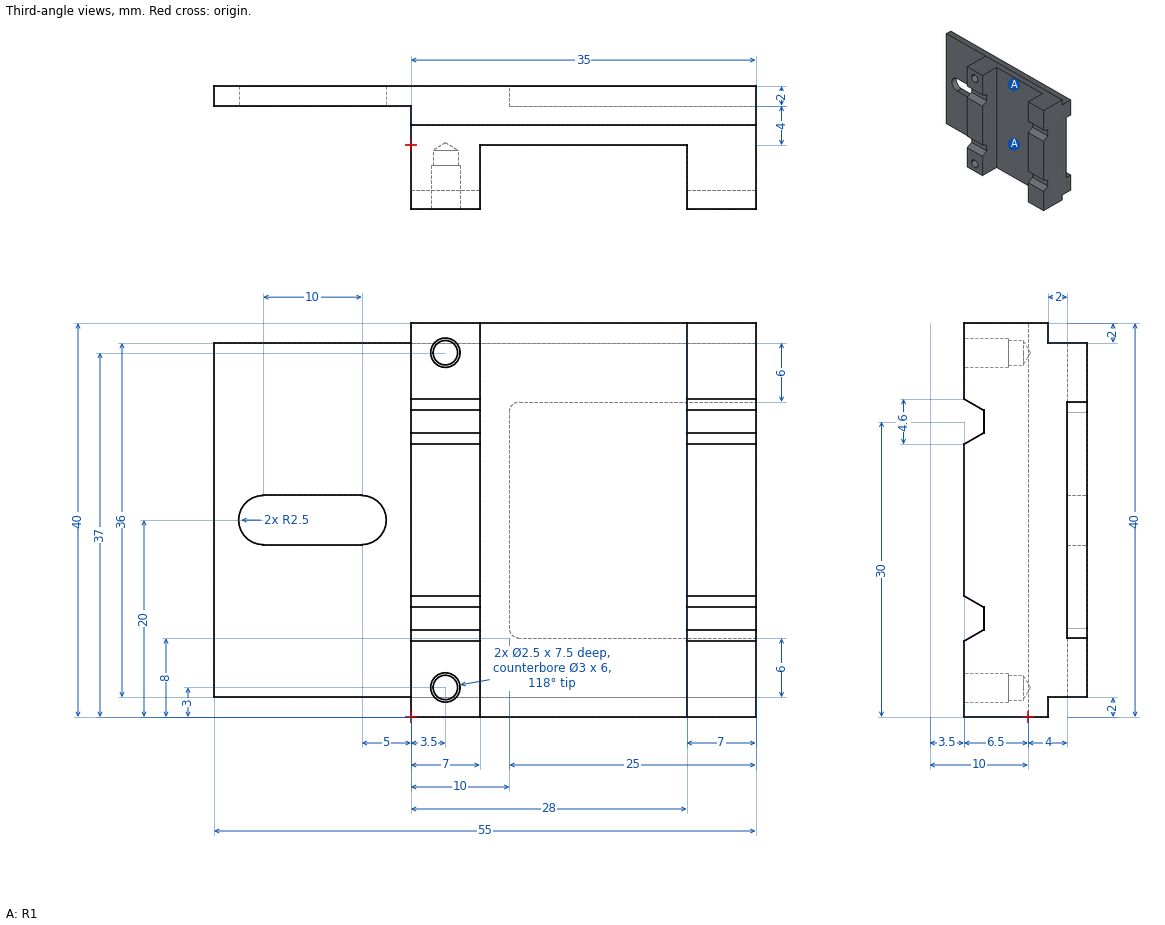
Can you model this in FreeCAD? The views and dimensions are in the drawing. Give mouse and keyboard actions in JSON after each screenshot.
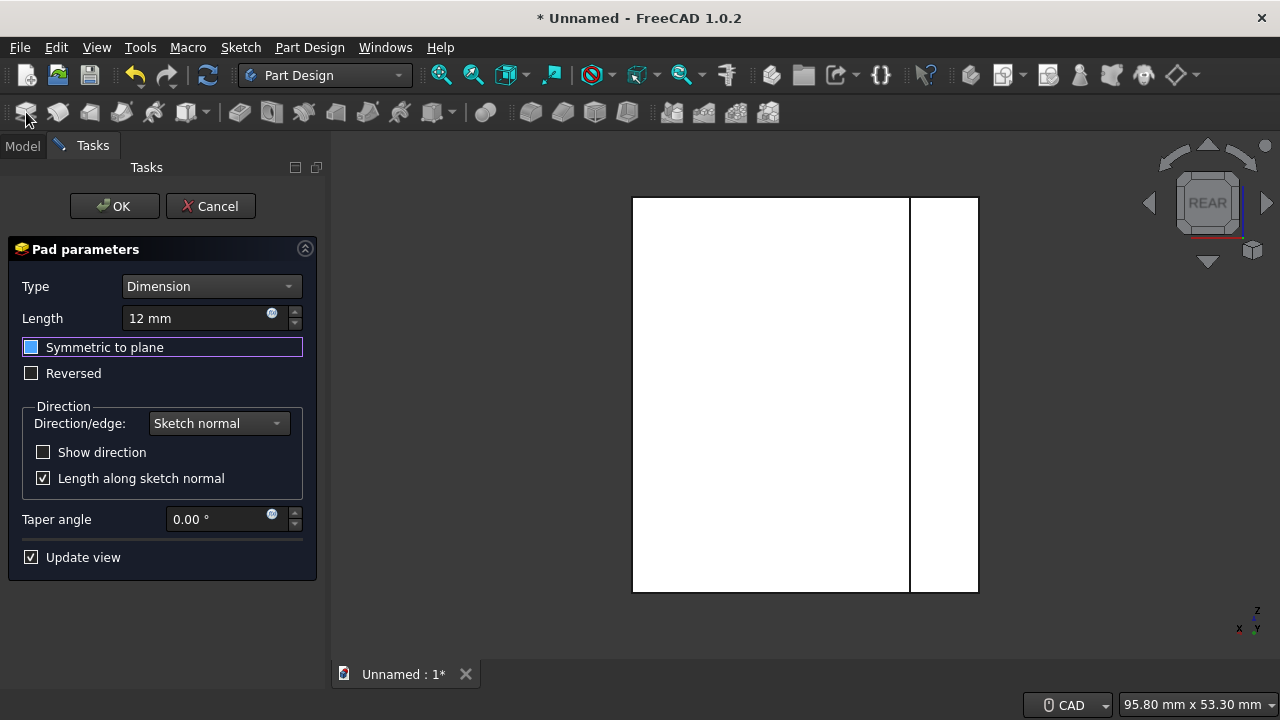
{"action": "left_click", "coordinate": [30, 373]}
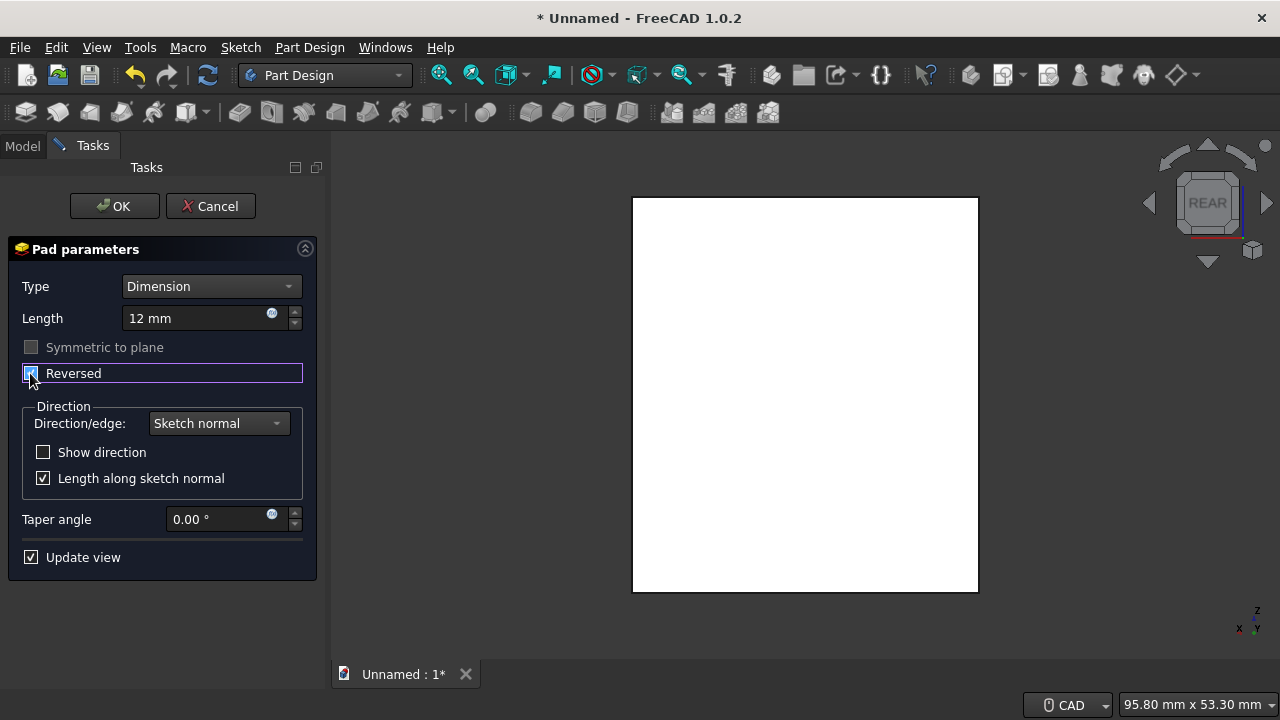
{"action": "left_click", "coordinate": [115, 206]}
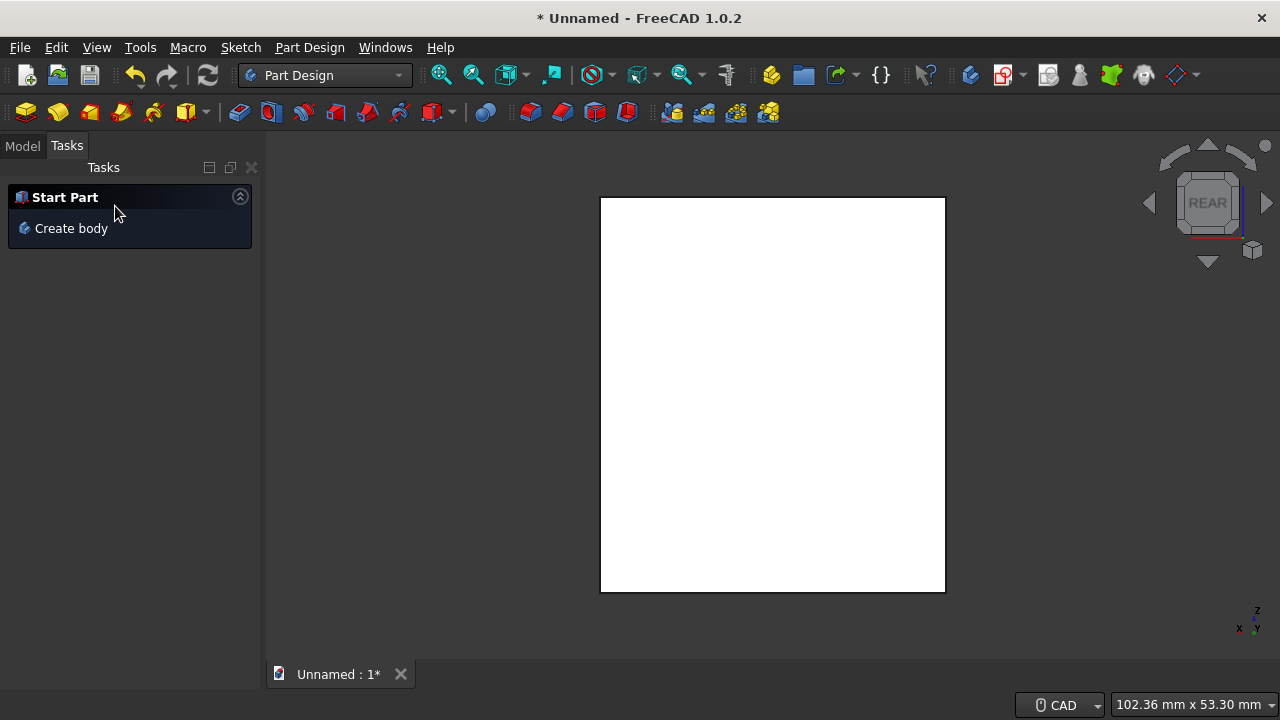
{"action": "key", "text": "0"}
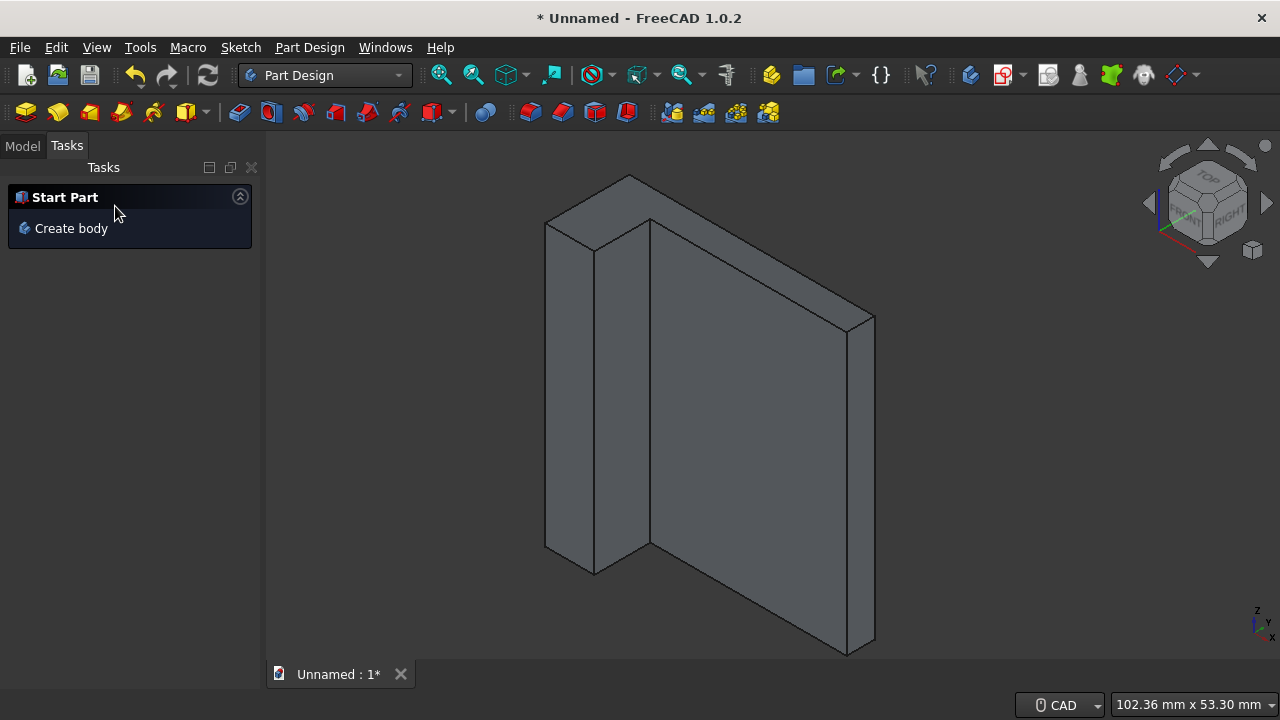
{"action": "left_click", "coordinate": [442, 76]}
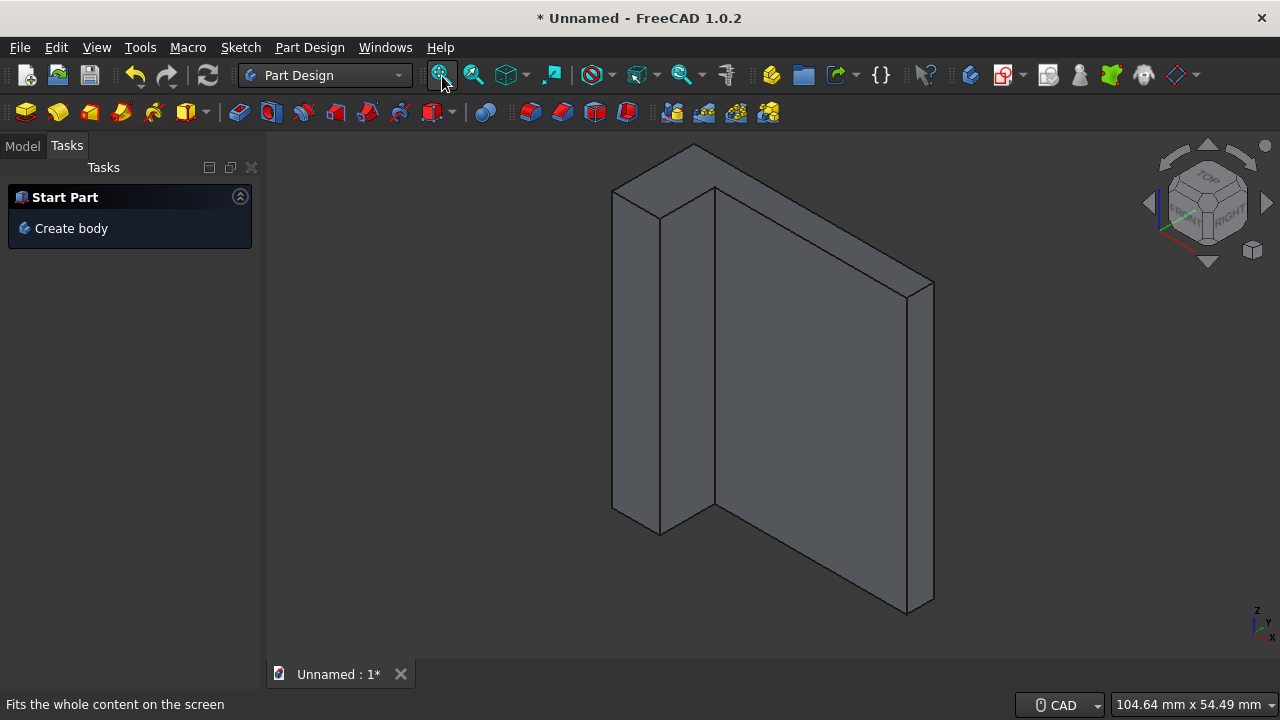
{"action": "left_click", "coordinate": [636, 272]}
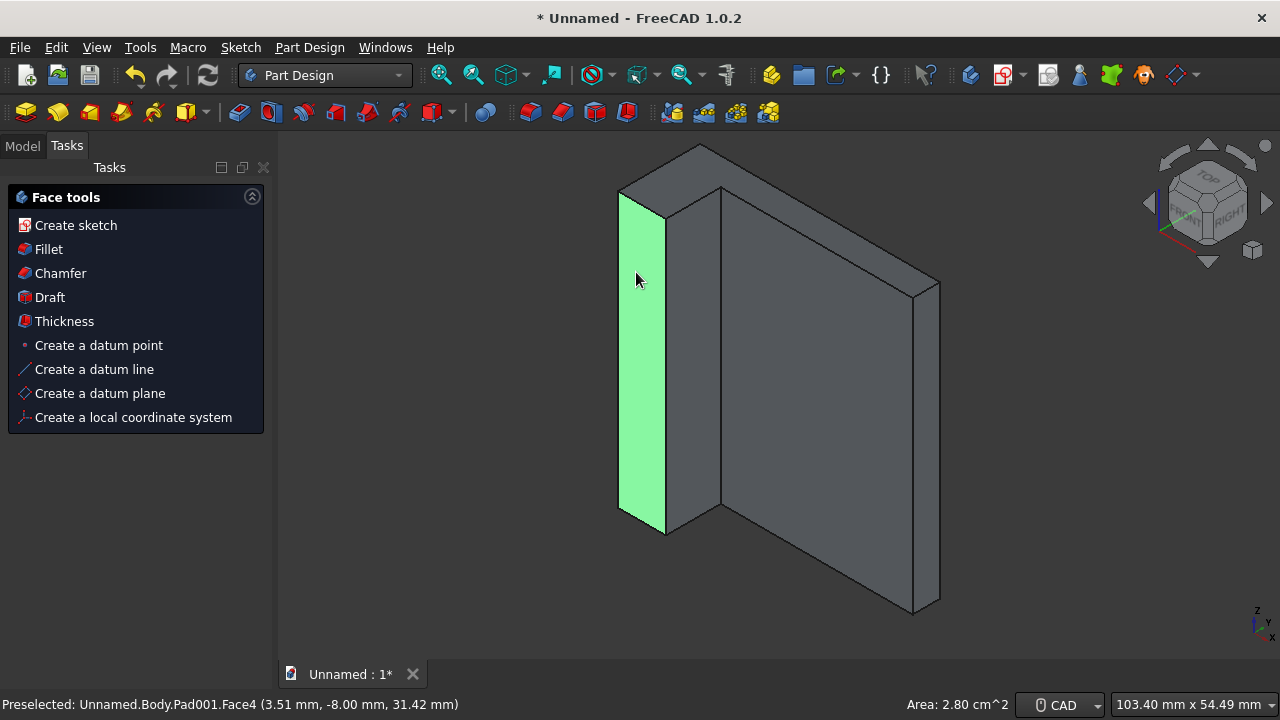
{"action": "left_click", "coordinate": [1004, 76]}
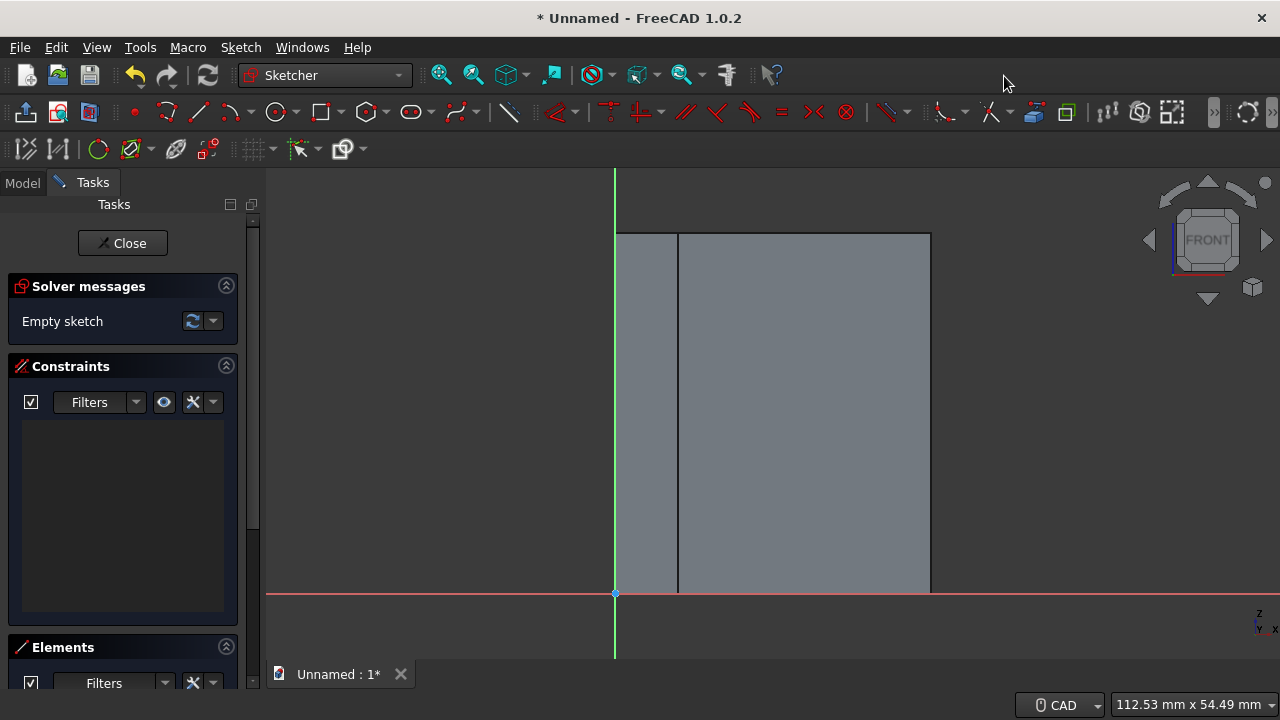
{"action": "left_click", "coordinate": [276, 112]}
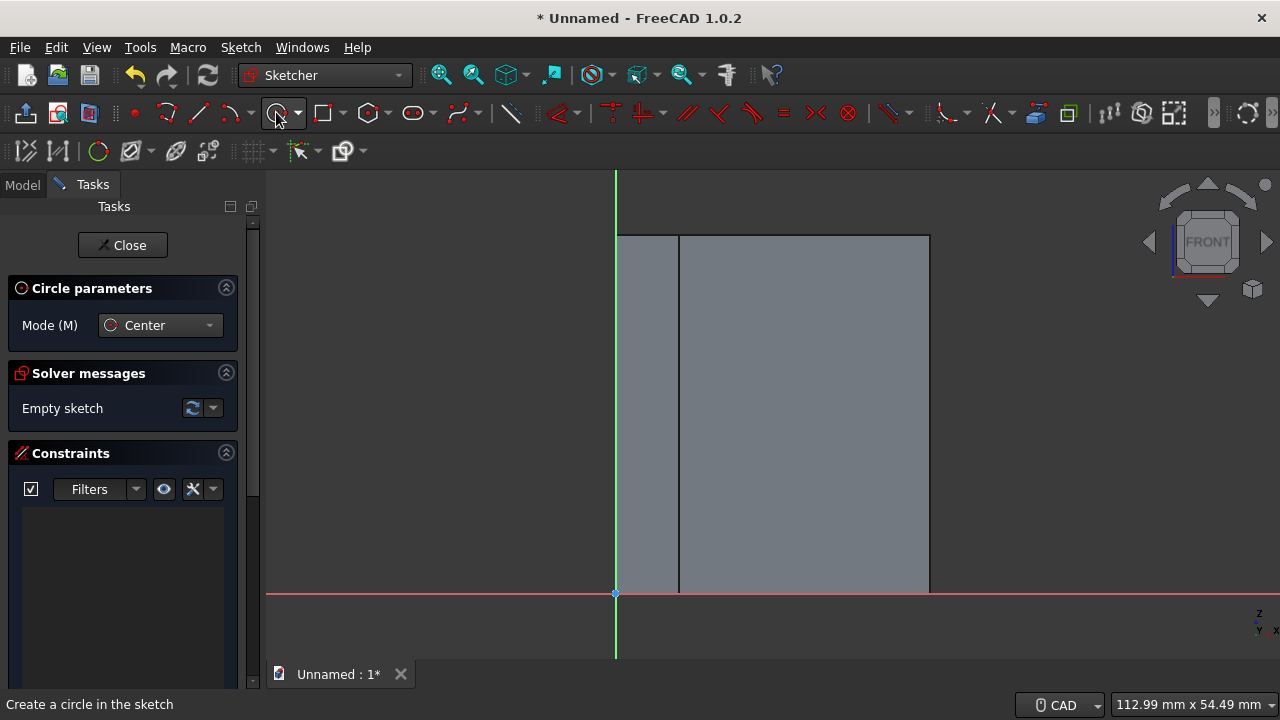
{"action": "scroll", "coordinate": [647, 567], "scroll_direction": "up", "scroll_amount": 4}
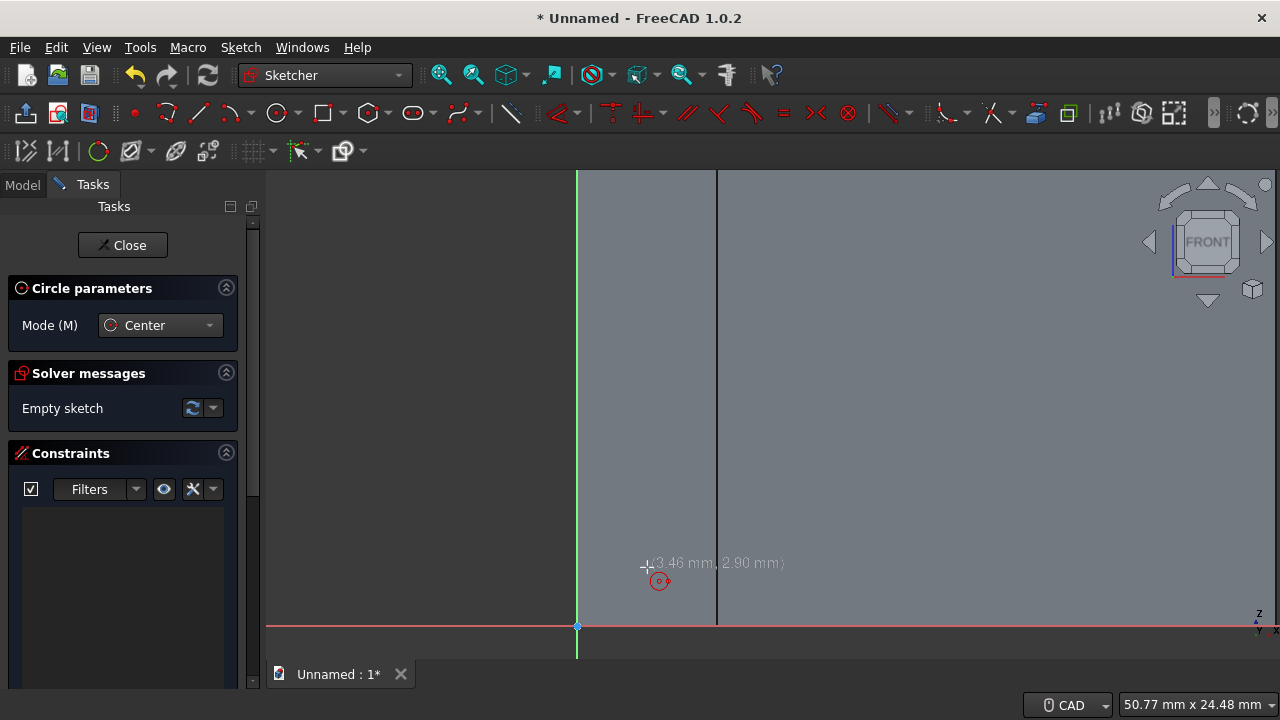
{"action": "left_click", "coordinate": [647, 566]}
{"action": "mouse_move", "coordinate": [665, 548]}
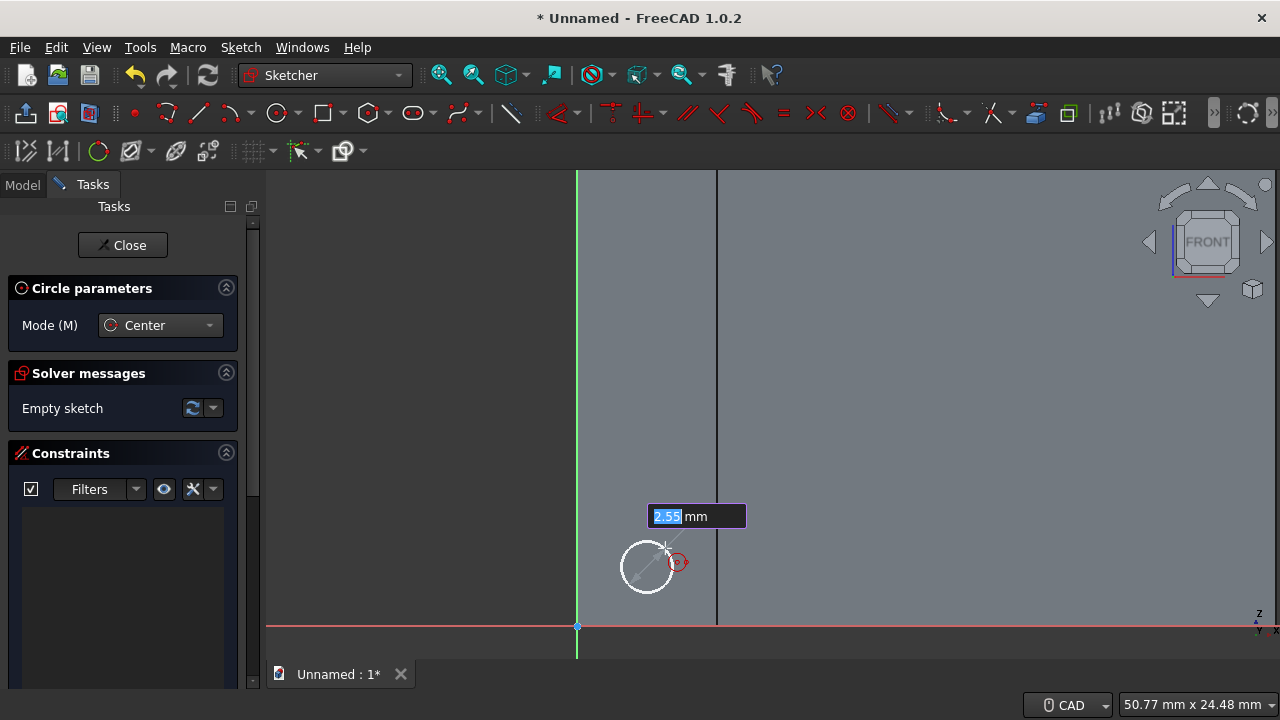
{"action": "type", "text": "2.5"}
{"action": "key", "text": "Return"}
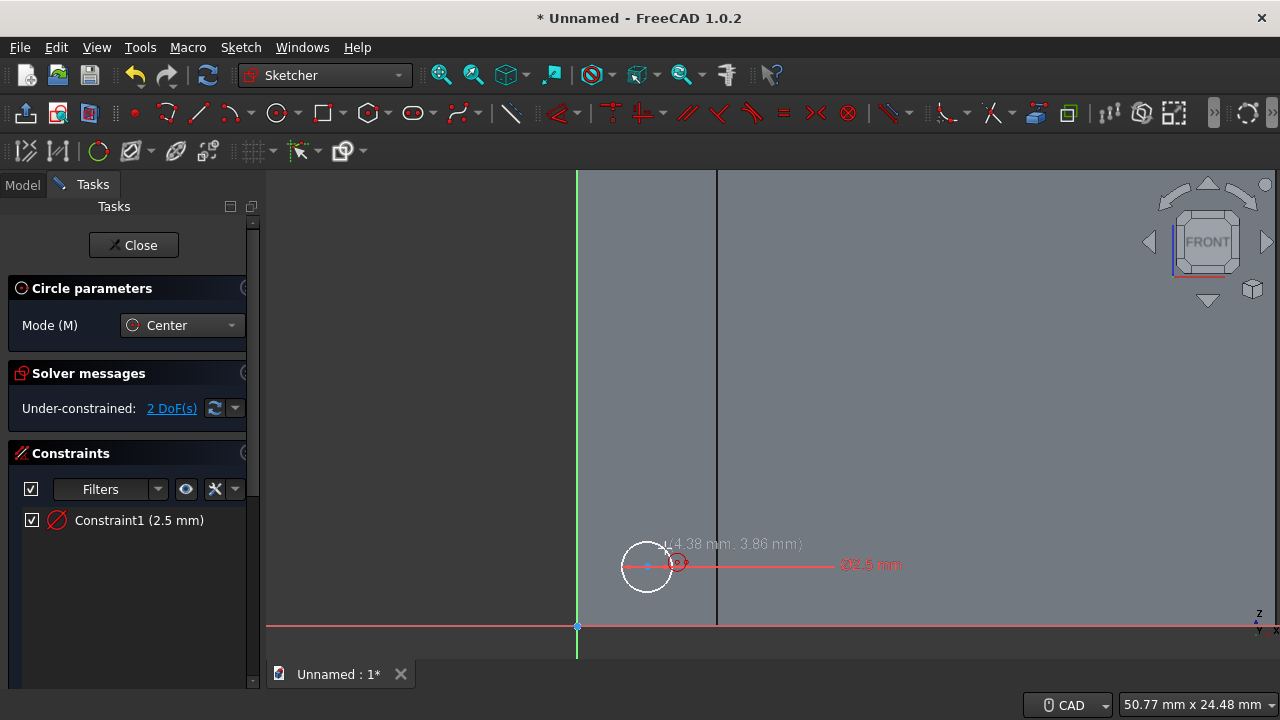
{"action": "scroll", "coordinate": [751, 514], "scroll_direction": "down", "scroll_amount": 5}